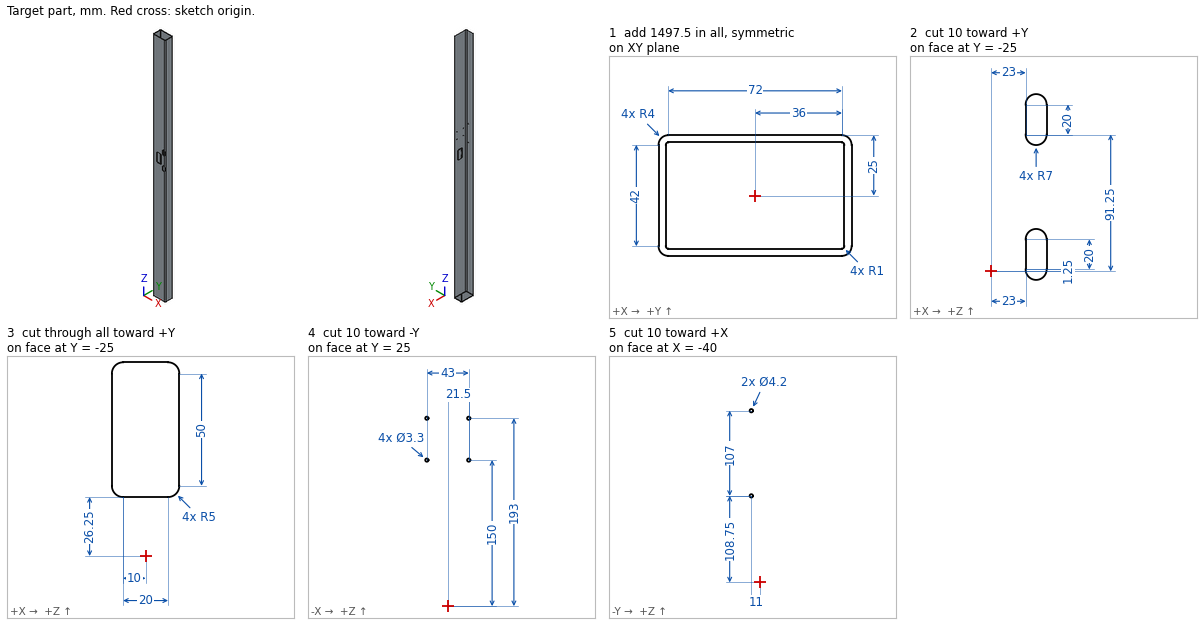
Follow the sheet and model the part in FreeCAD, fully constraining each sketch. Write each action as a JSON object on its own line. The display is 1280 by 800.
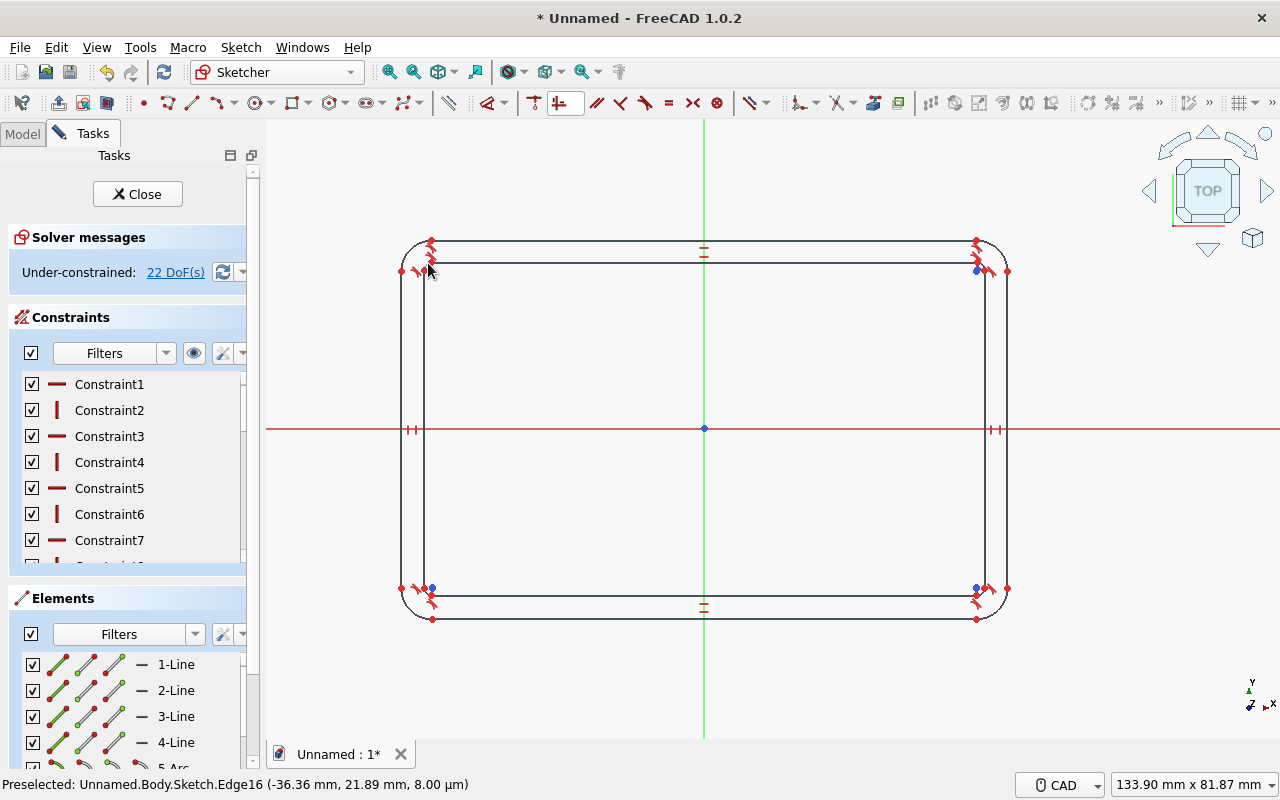
{"action": "left_click", "coordinate": [985, 366]}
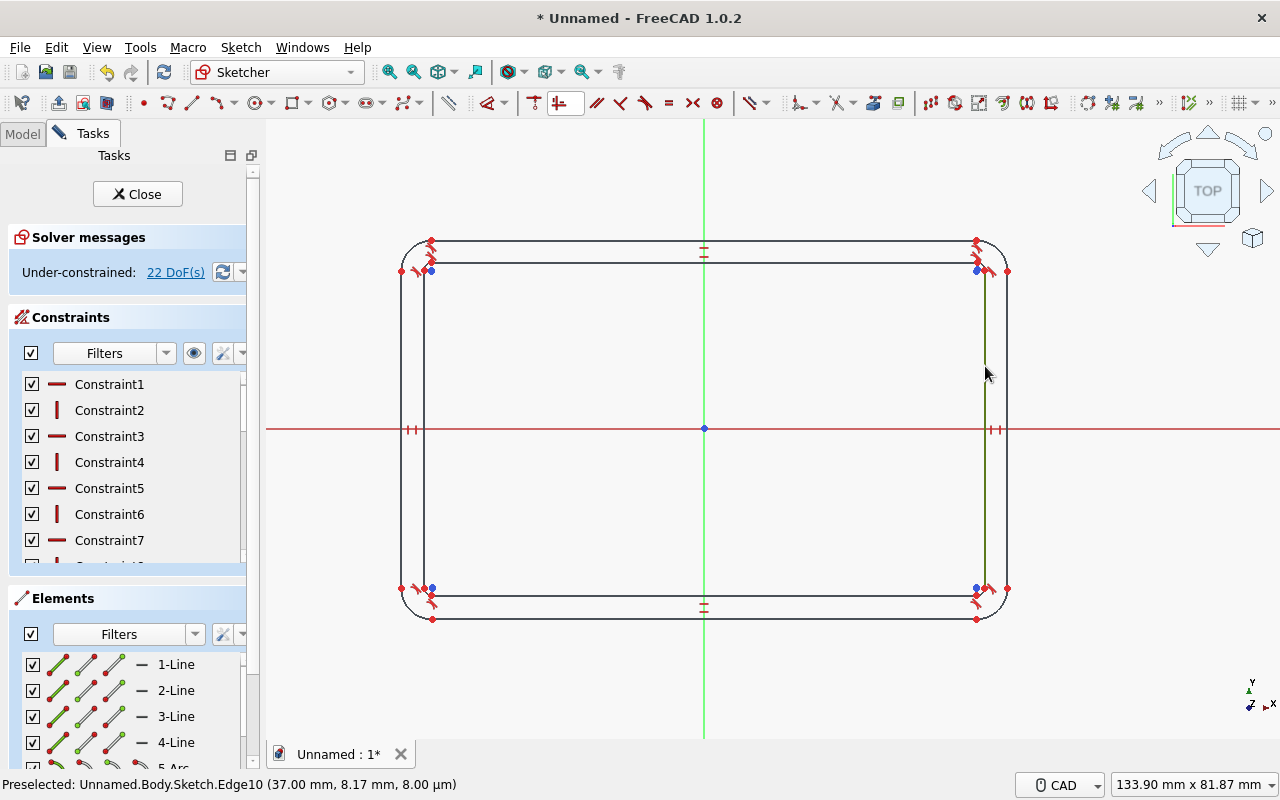
{"action": "scroll", "coordinate": [983, 265], "scroll_direction": "up", "scroll_amount": 5}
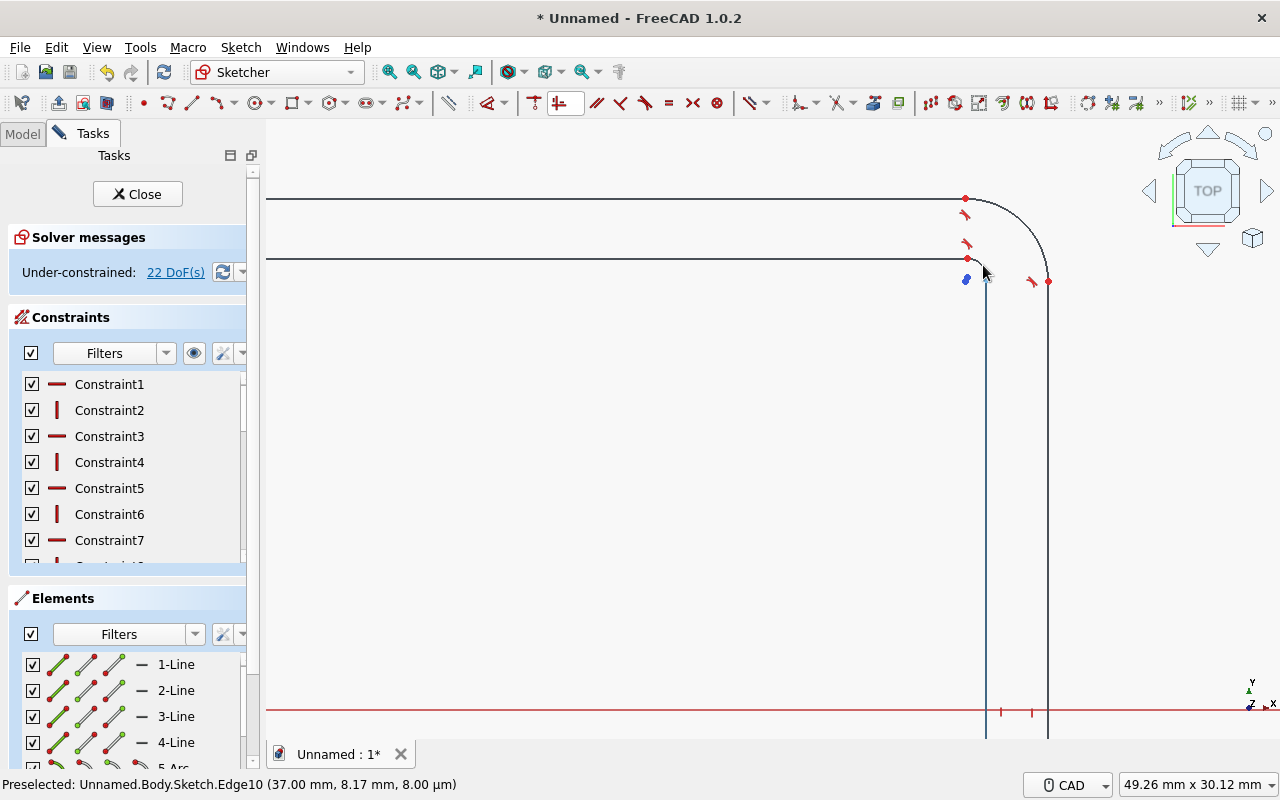
{"action": "left_click", "coordinate": [982, 265]}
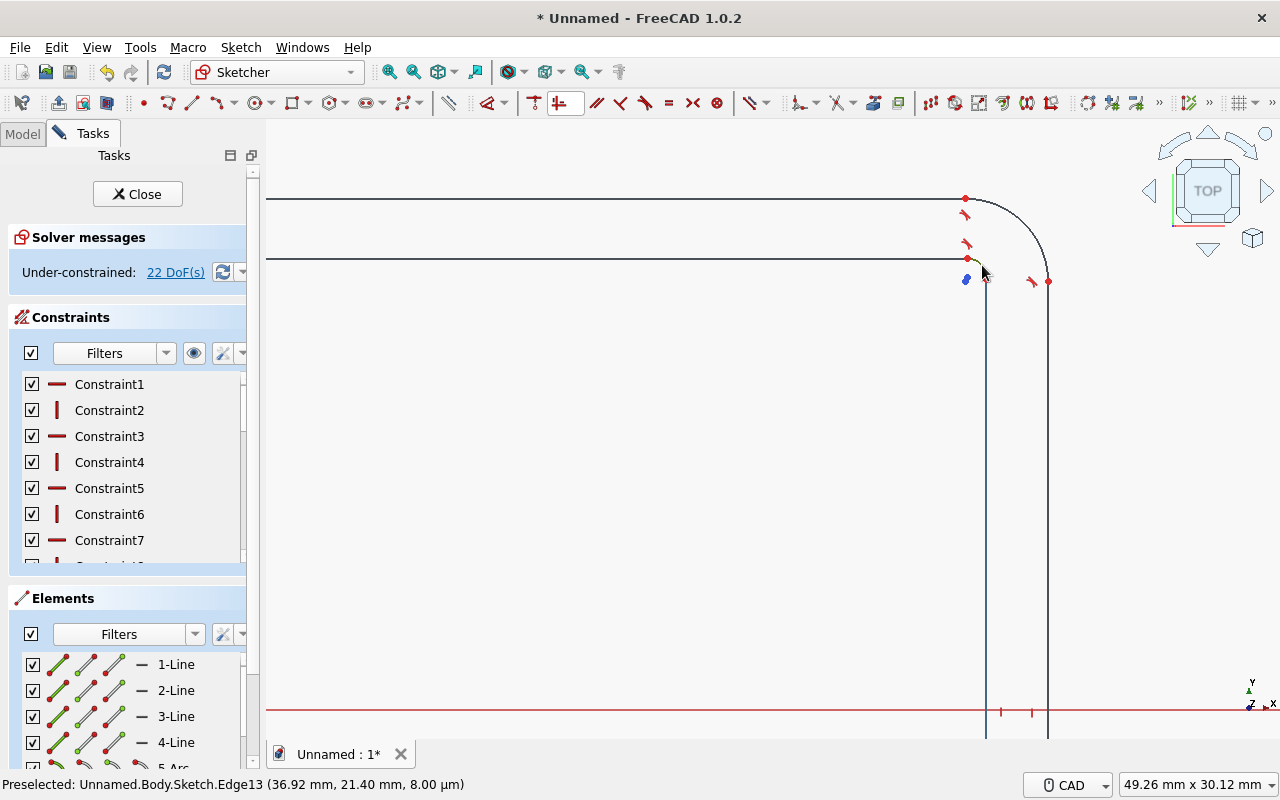
{"action": "key", "text": "t"}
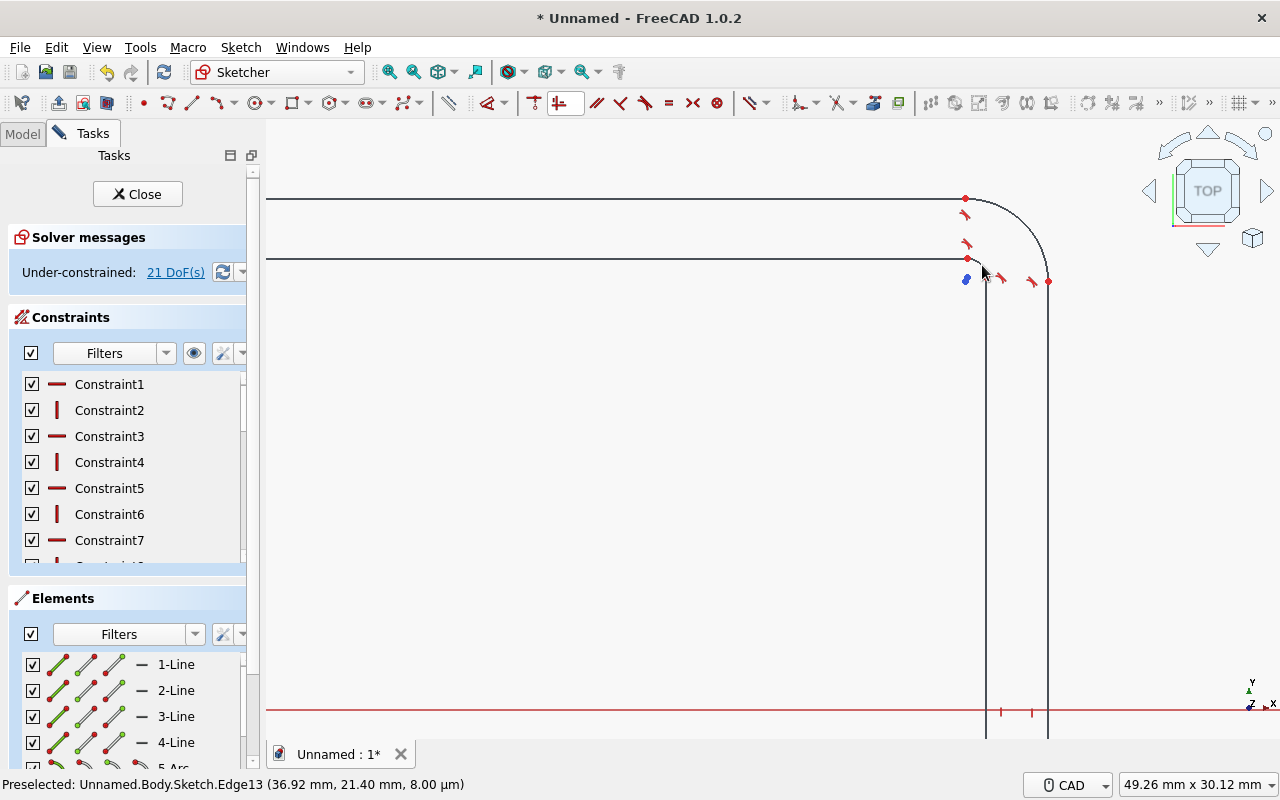
{"action": "left_click", "coordinate": [986, 538]}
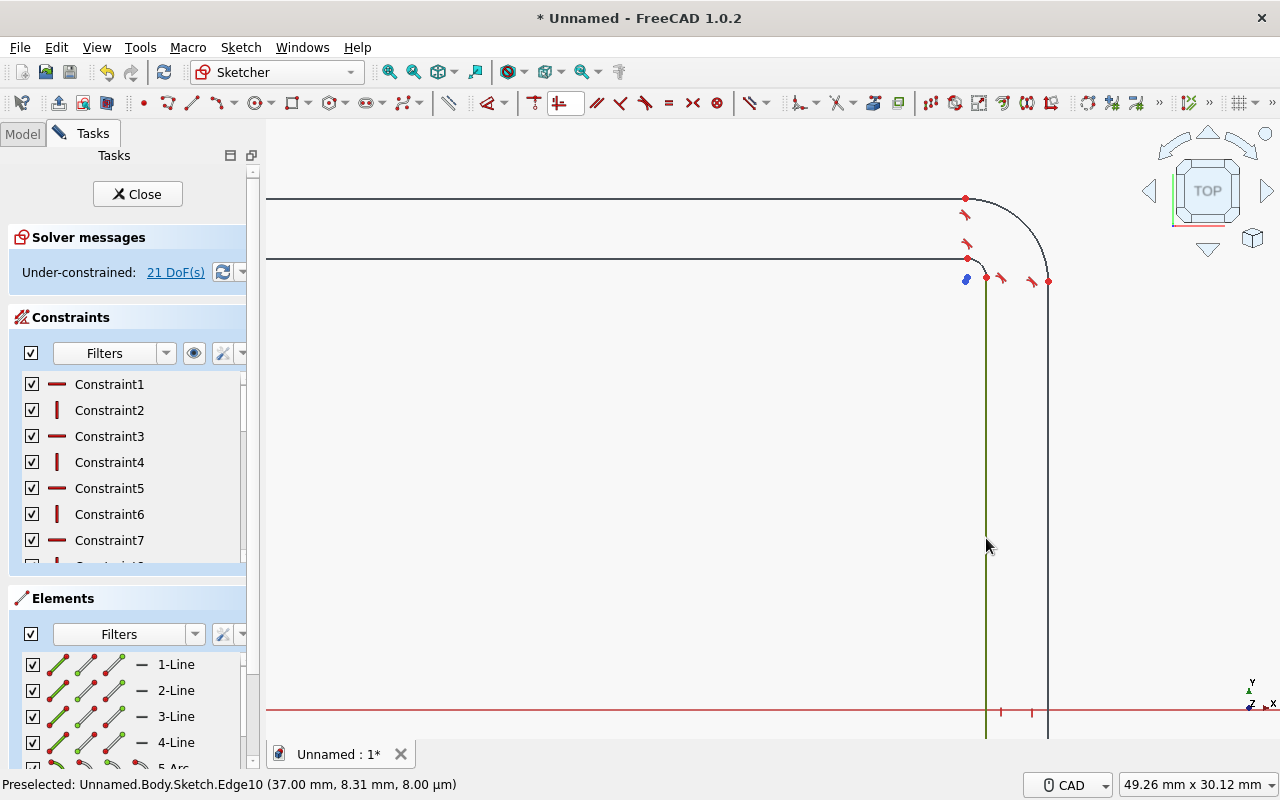
{"action": "scroll", "coordinate": [984, 265], "scroll_direction": "down", "scroll_amount": 5}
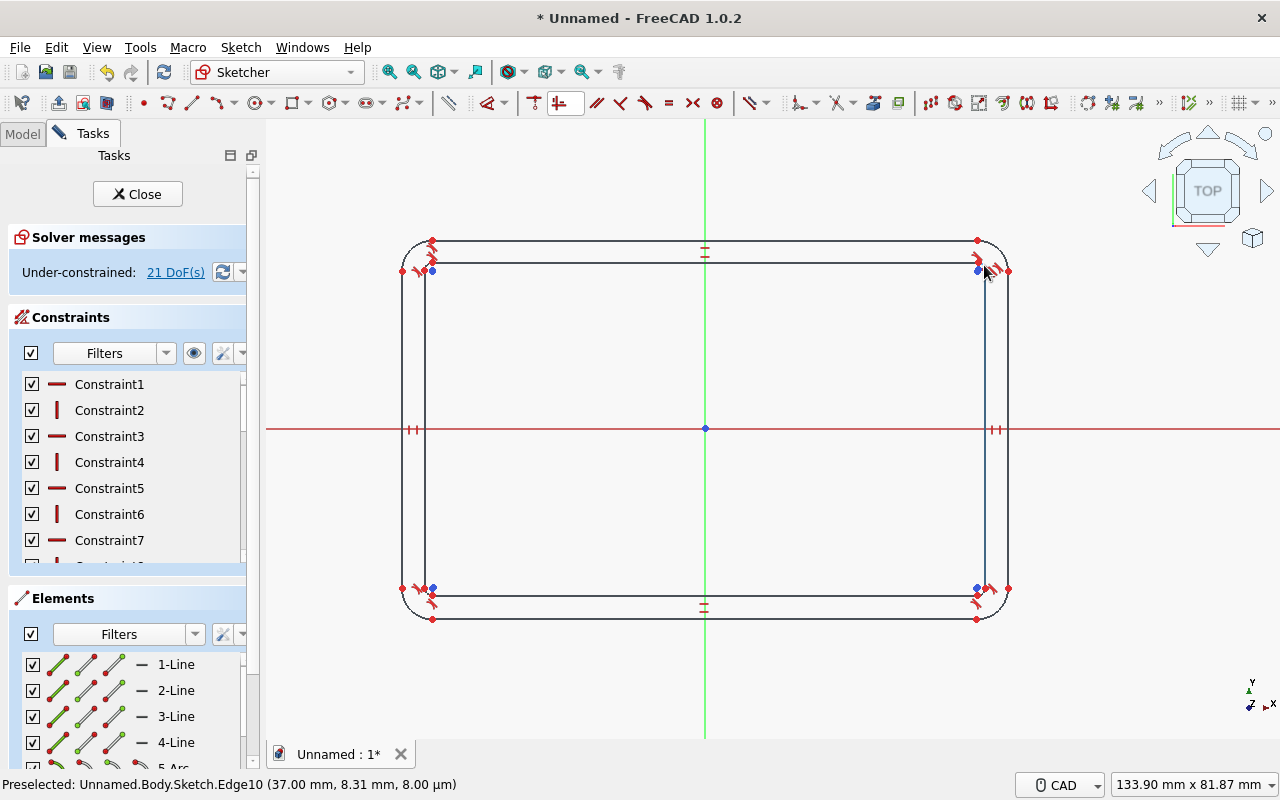
{"action": "scroll", "coordinate": [981, 595], "scroll_direction": "up", "scroll_amount": 7}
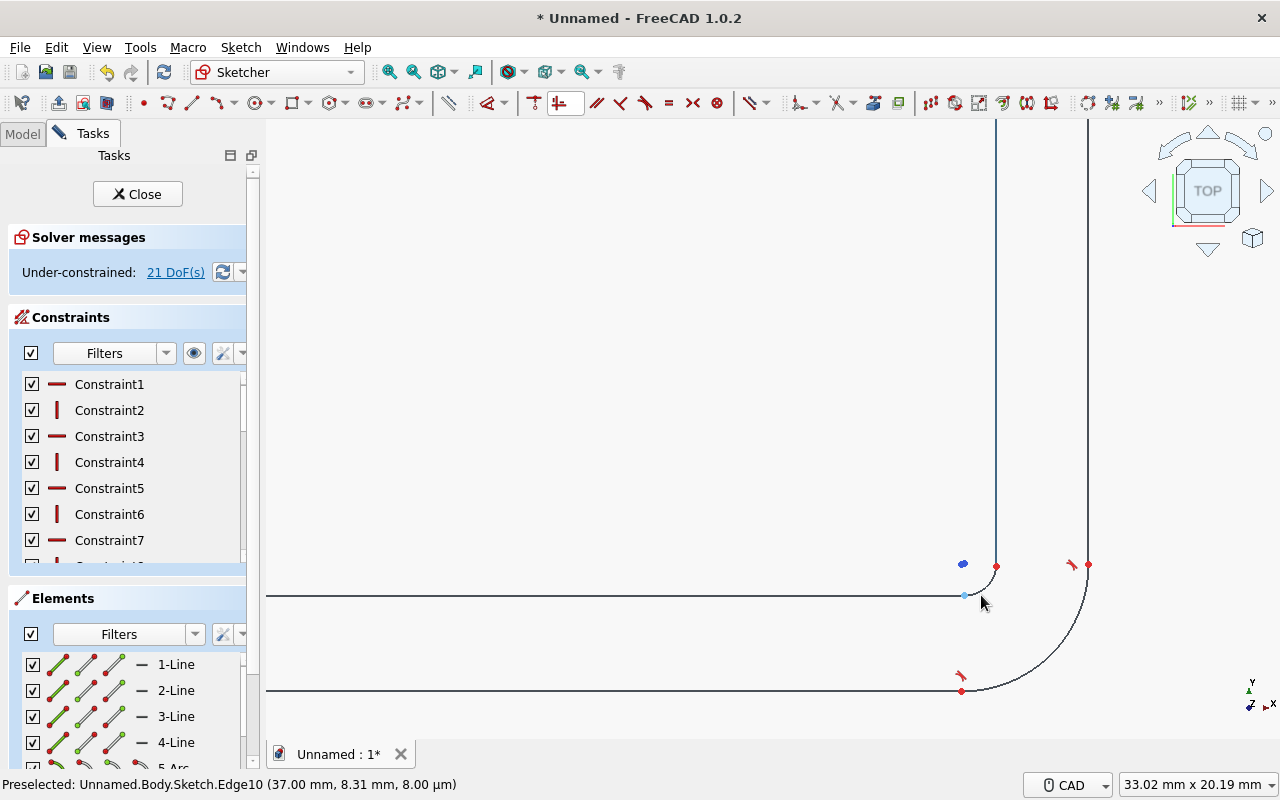
{"action": "left_click", "coordinate": [979, 592]}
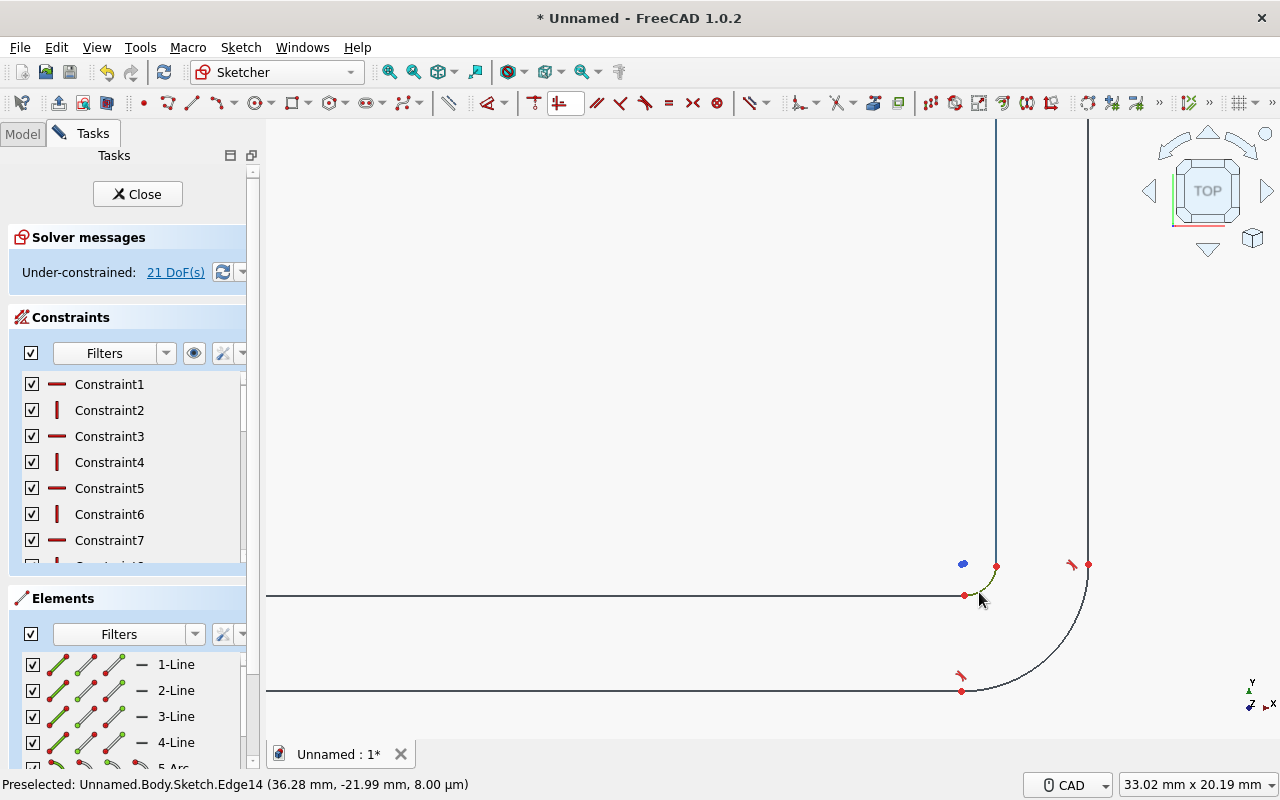
{"action": "key", "text": "t"}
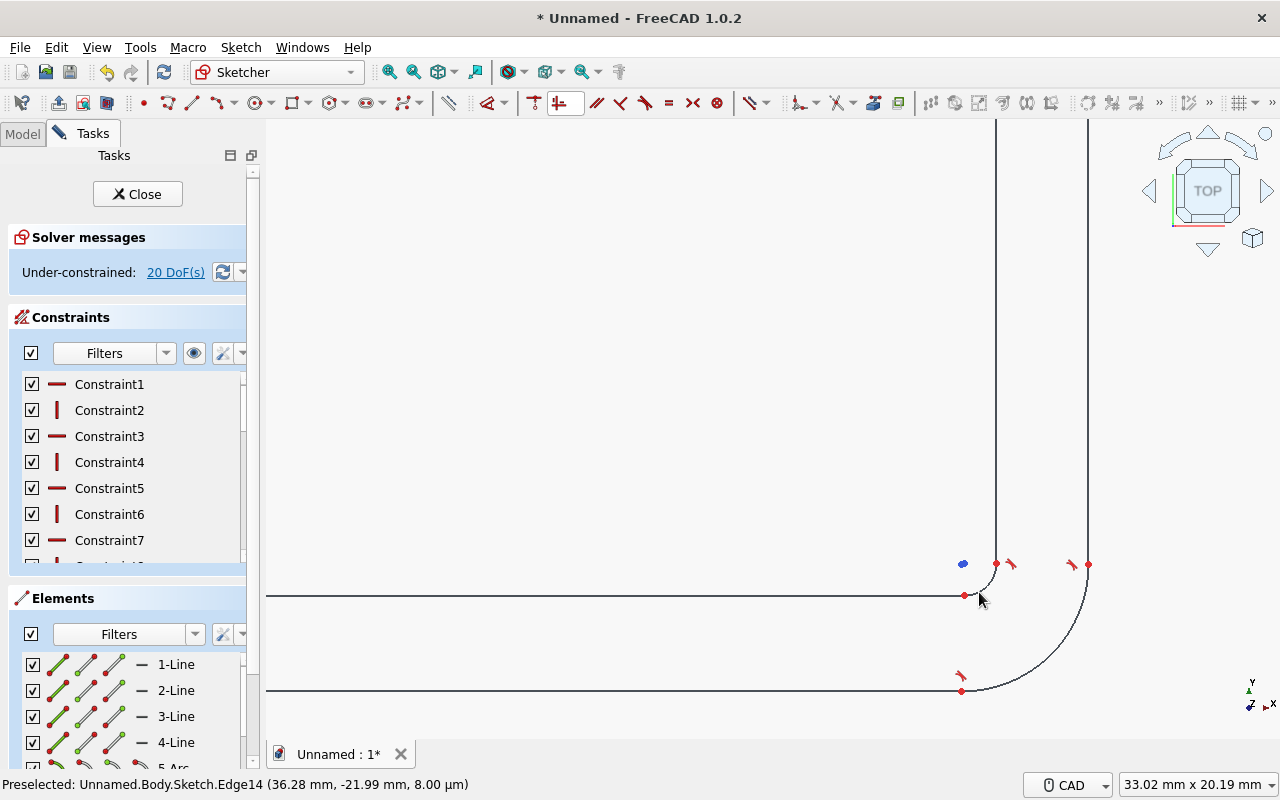
{"action": "scroll", "coordinate": [981, 596], "scroll_direction": "down", "scroll_amount": 7}